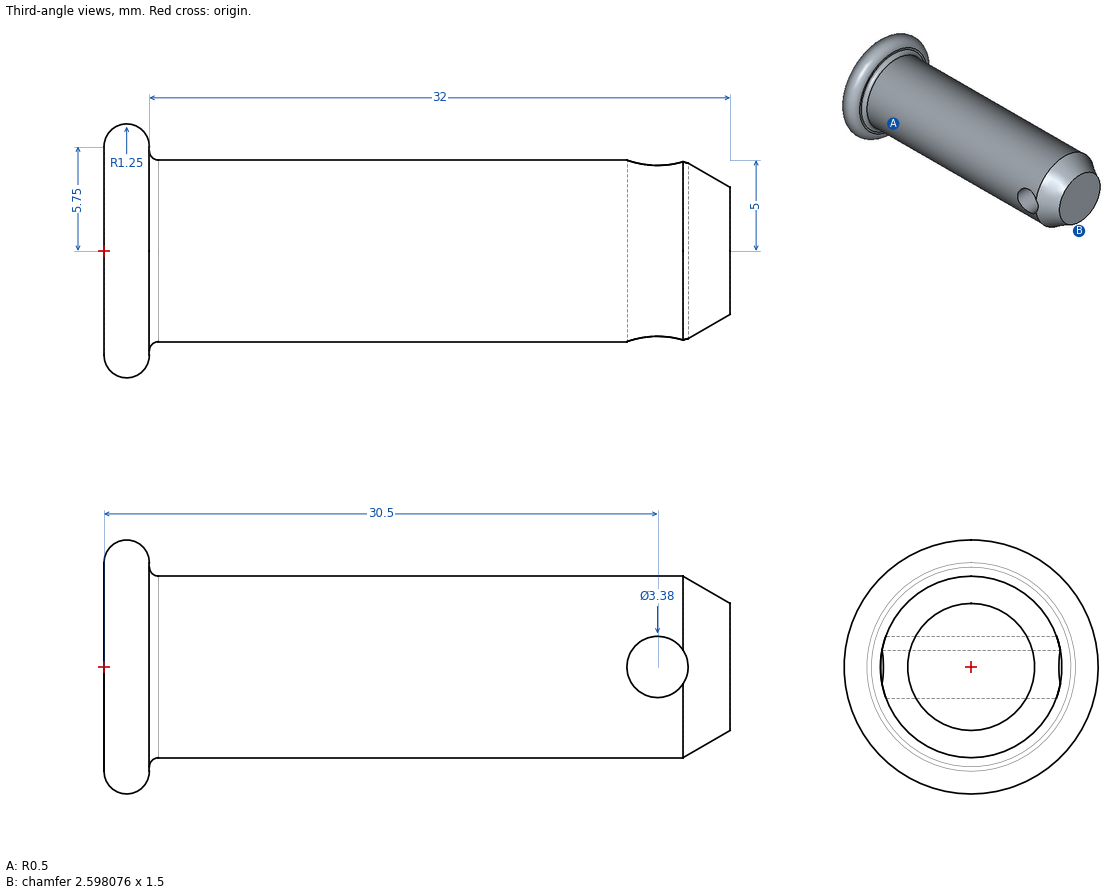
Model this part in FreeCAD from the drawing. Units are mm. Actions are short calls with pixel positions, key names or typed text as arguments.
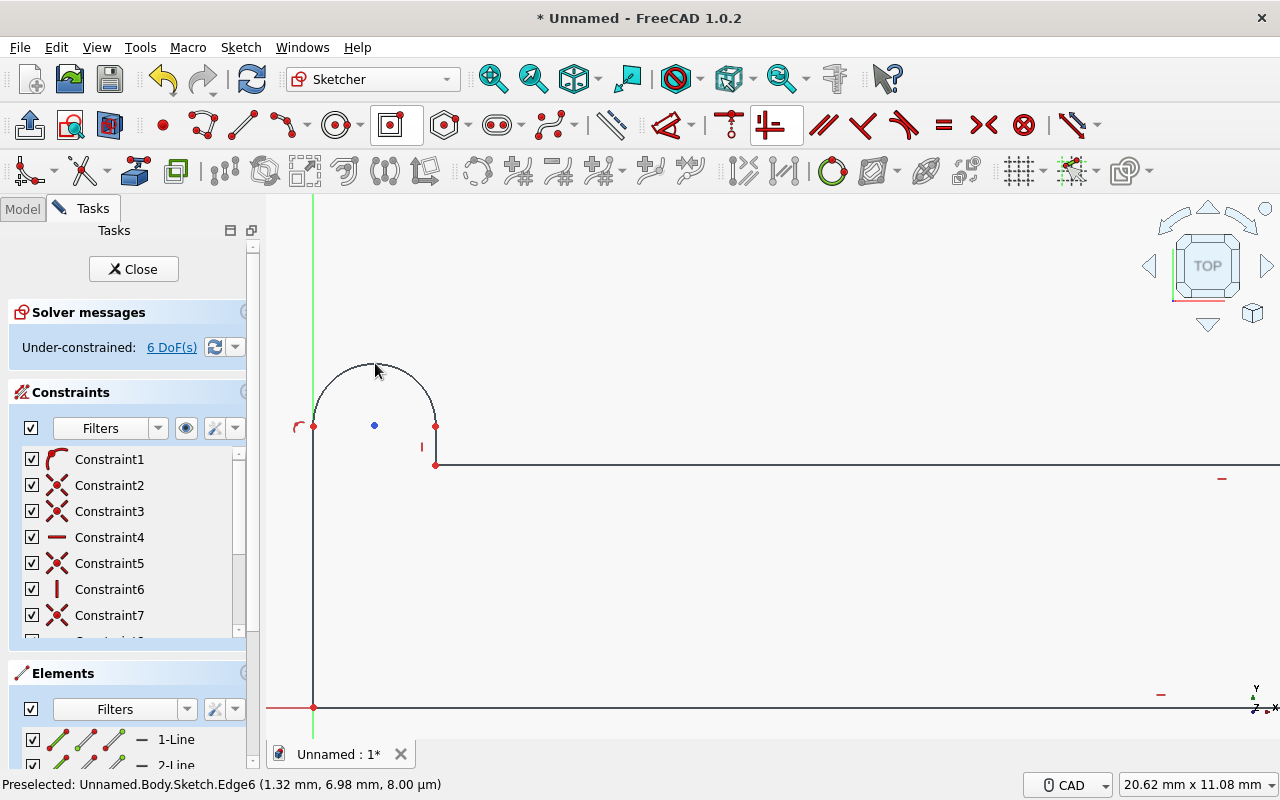
click(313, 511)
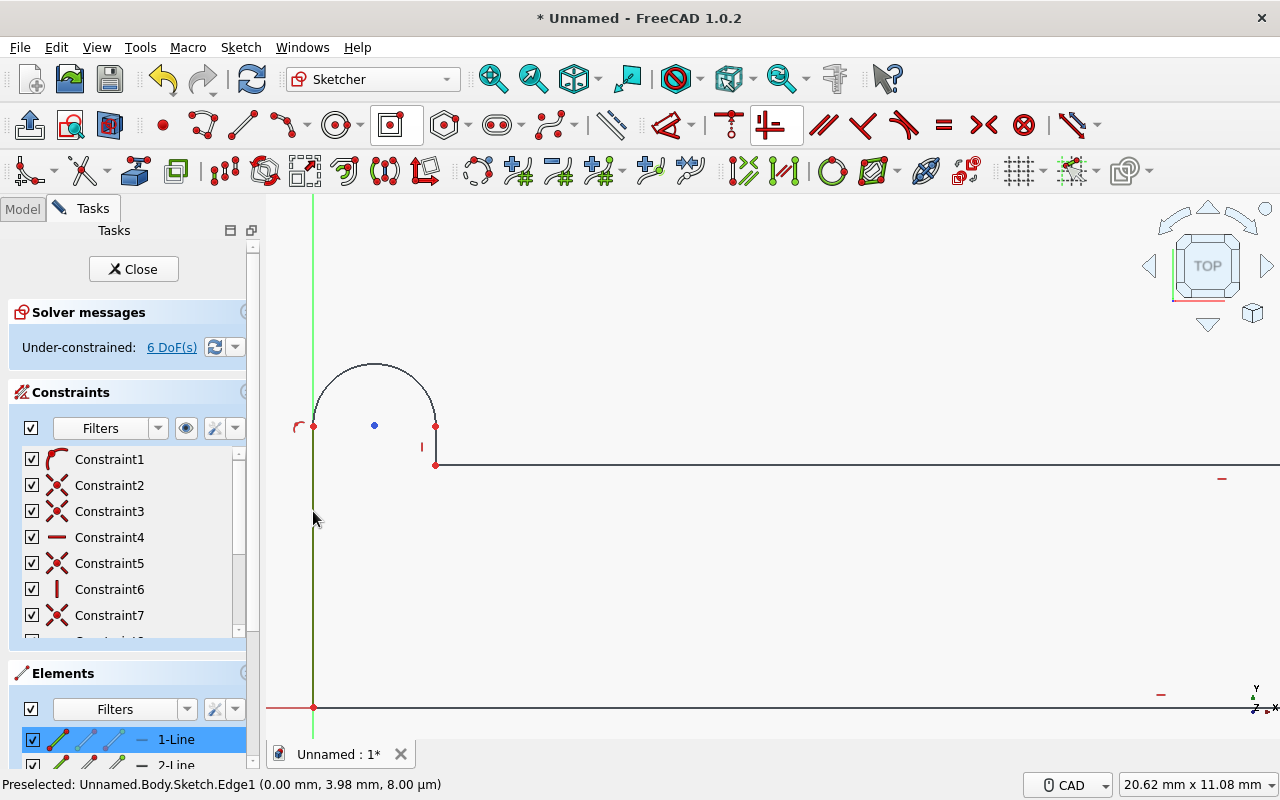
click(411, 376)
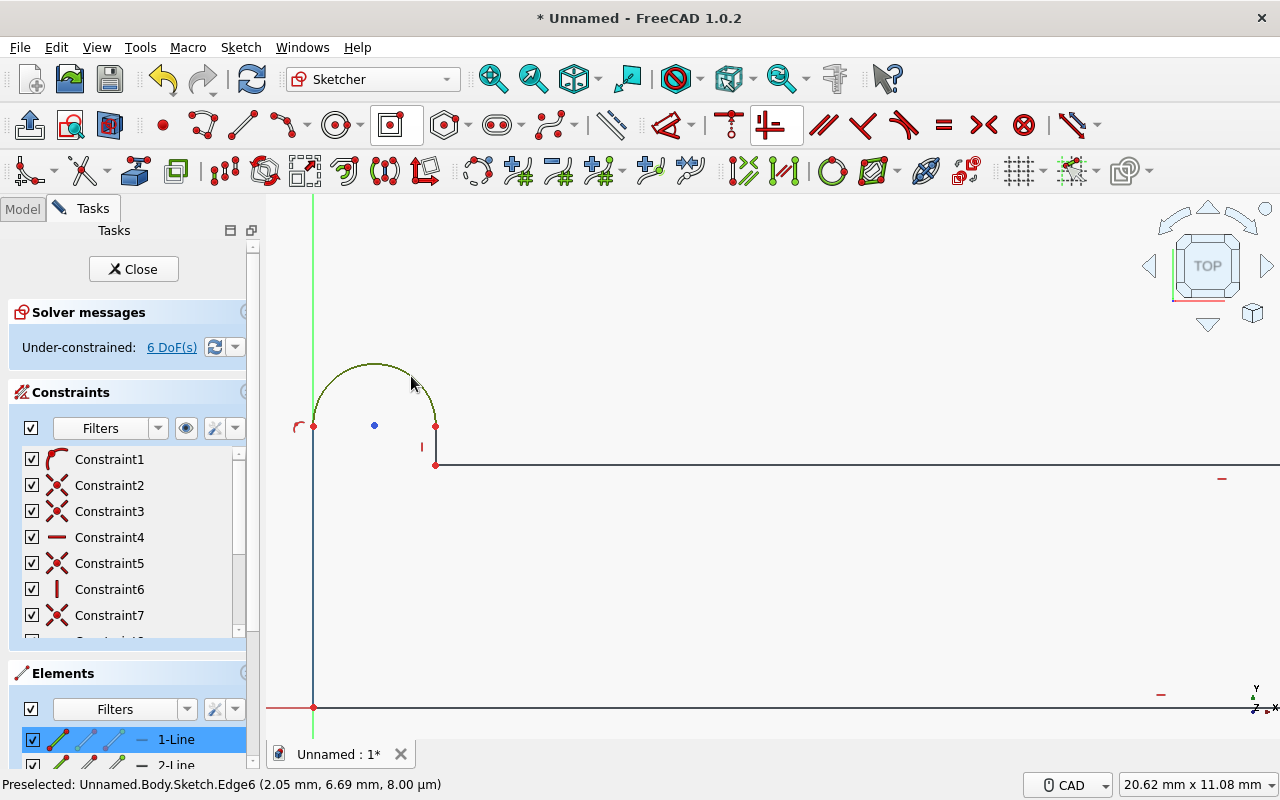
key(t)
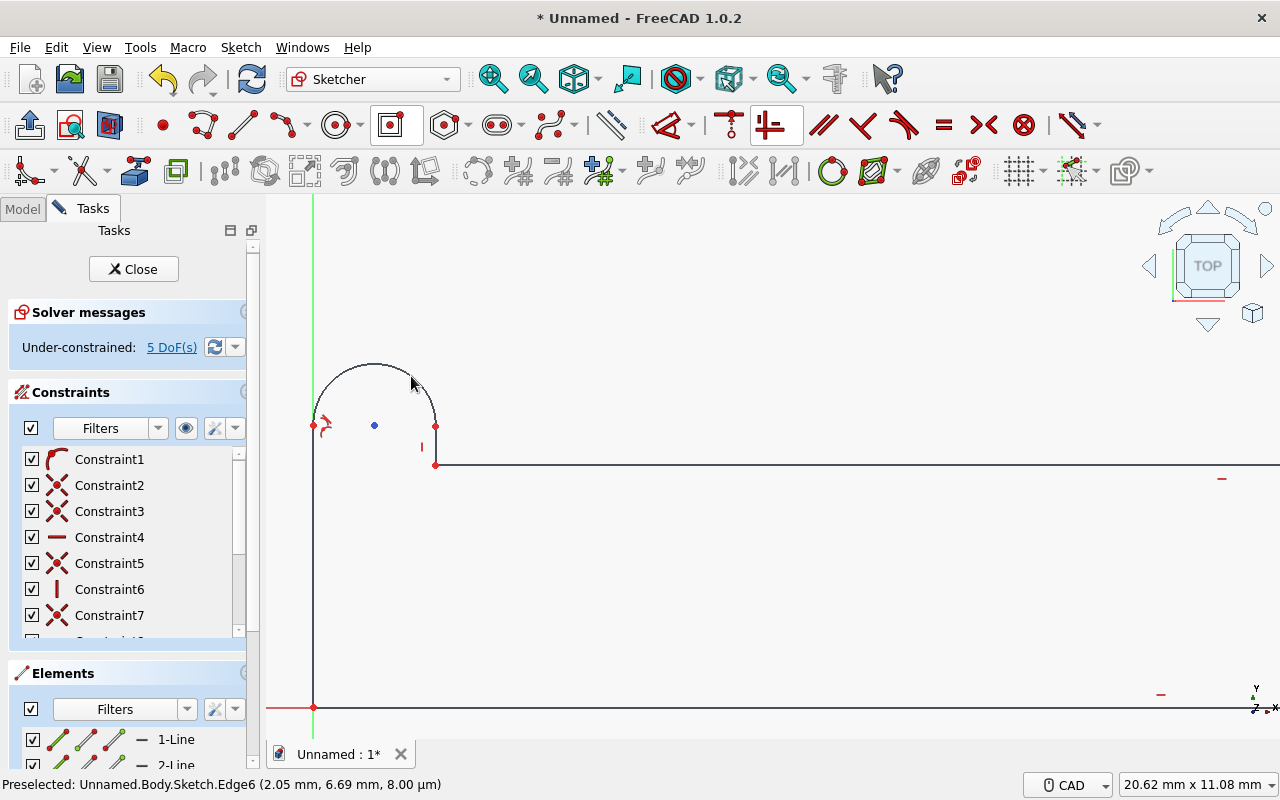
click(436, 454)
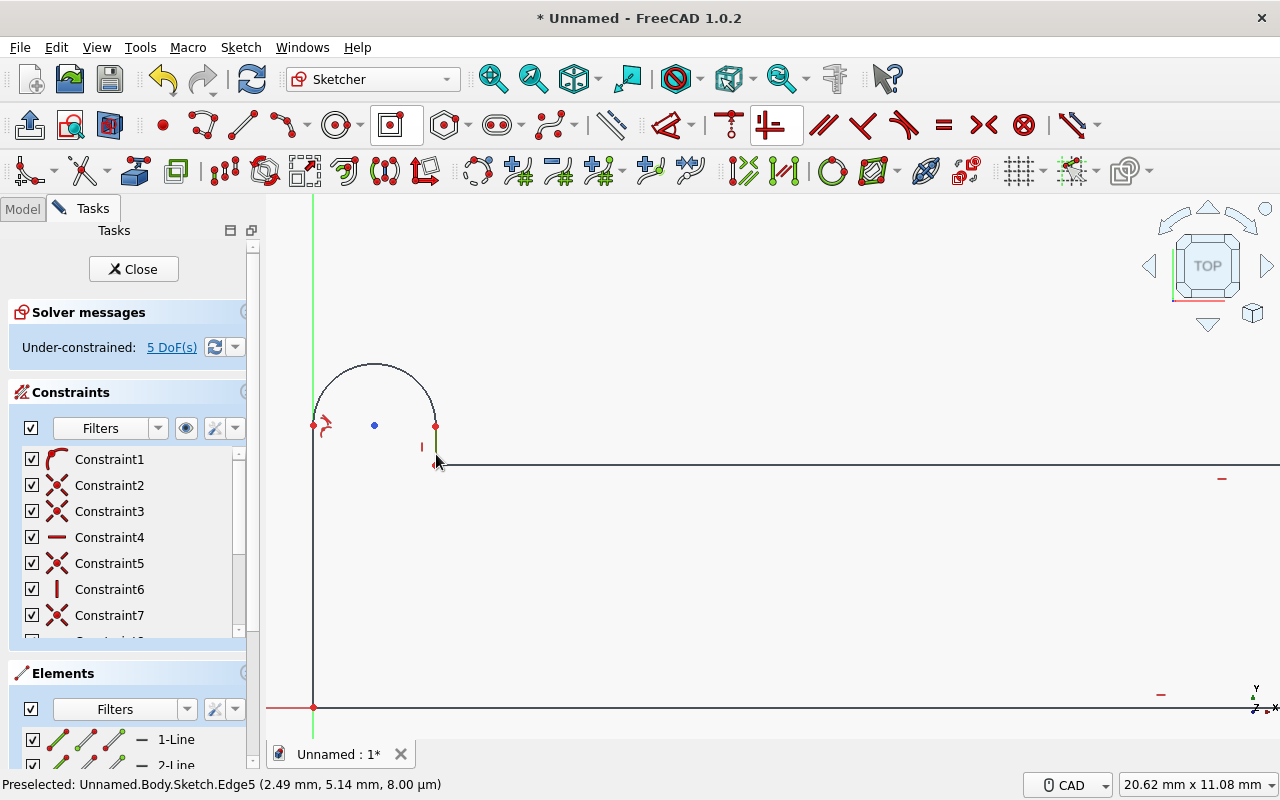
click(411, 376)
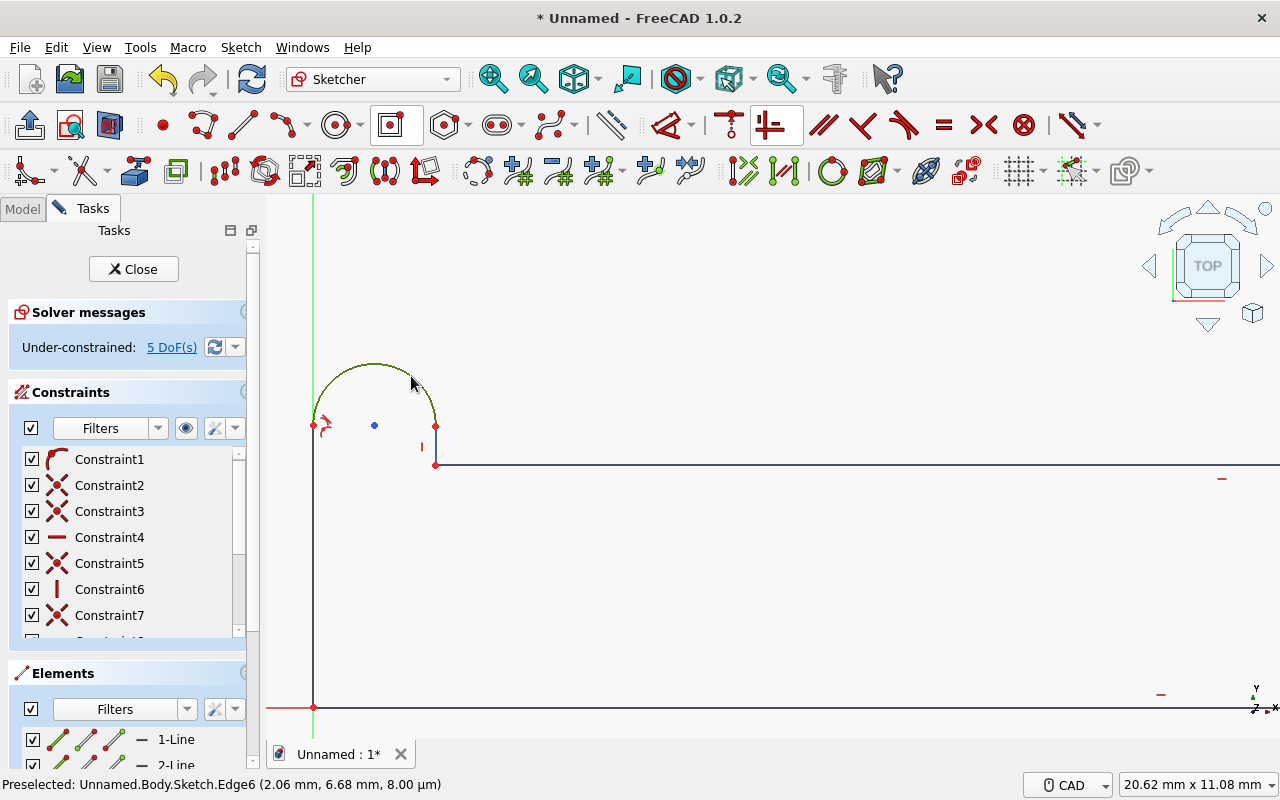
key(t)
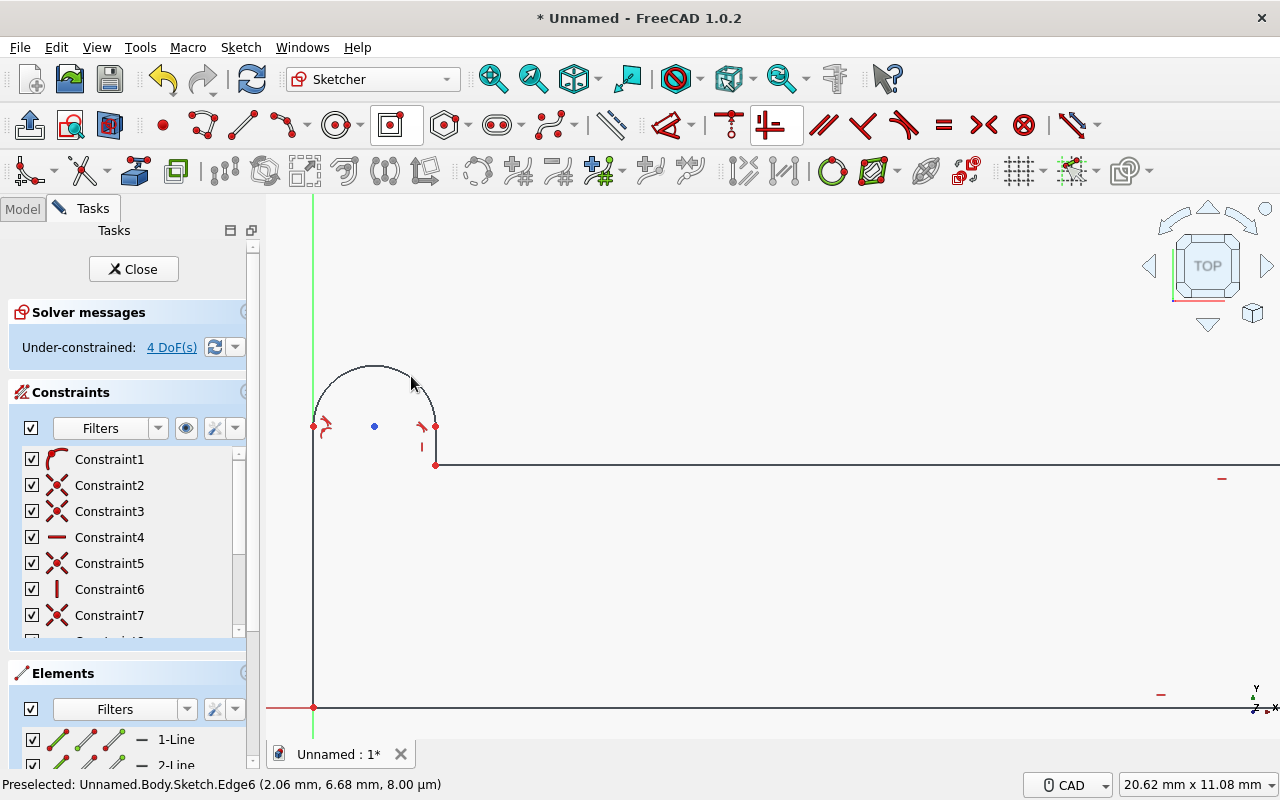
click(410, 377)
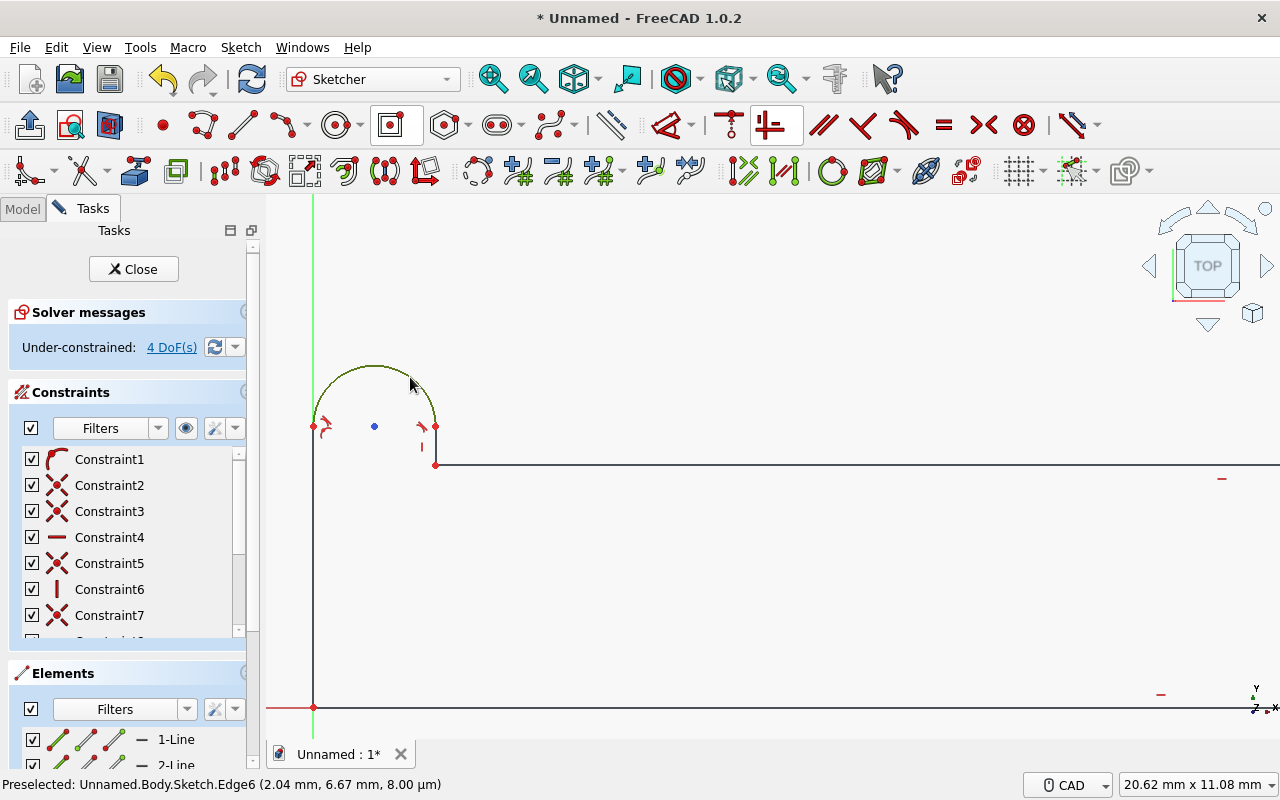
key(k)
key(r)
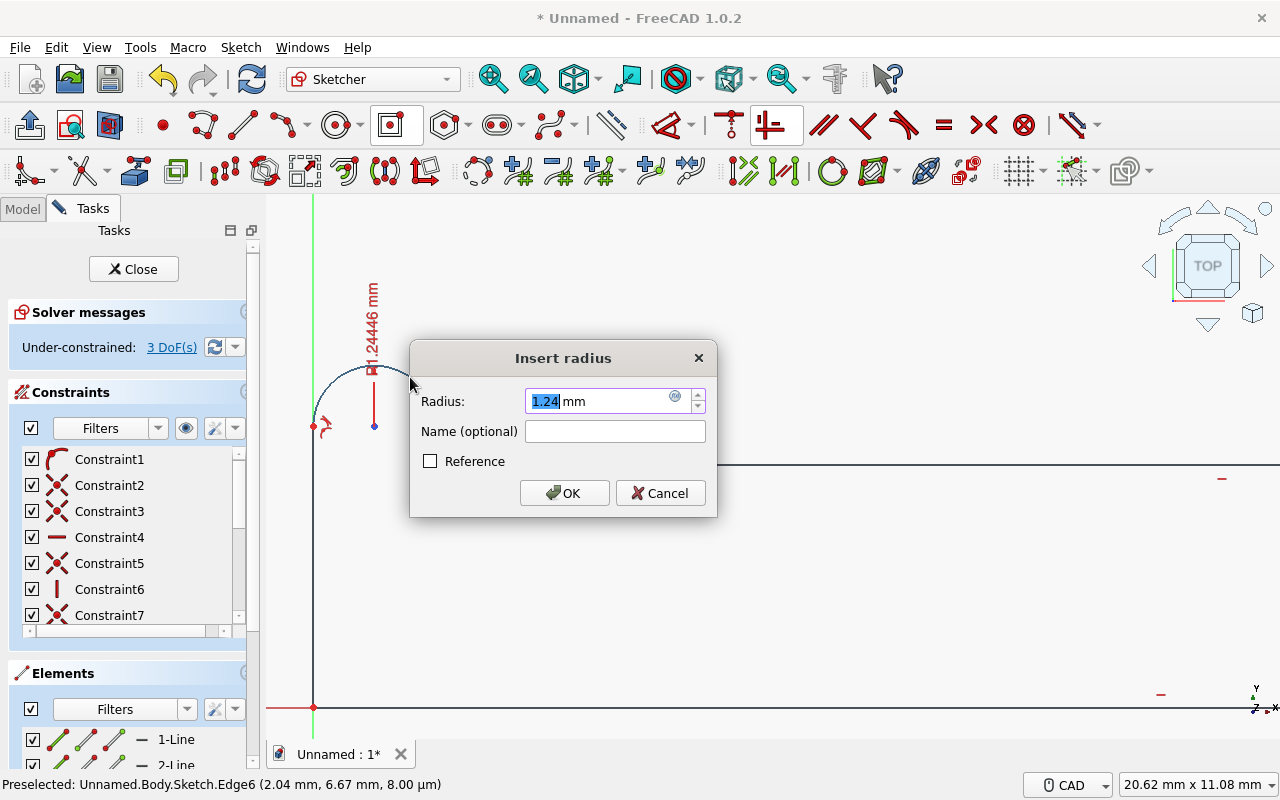
text(1.25)
key(Return)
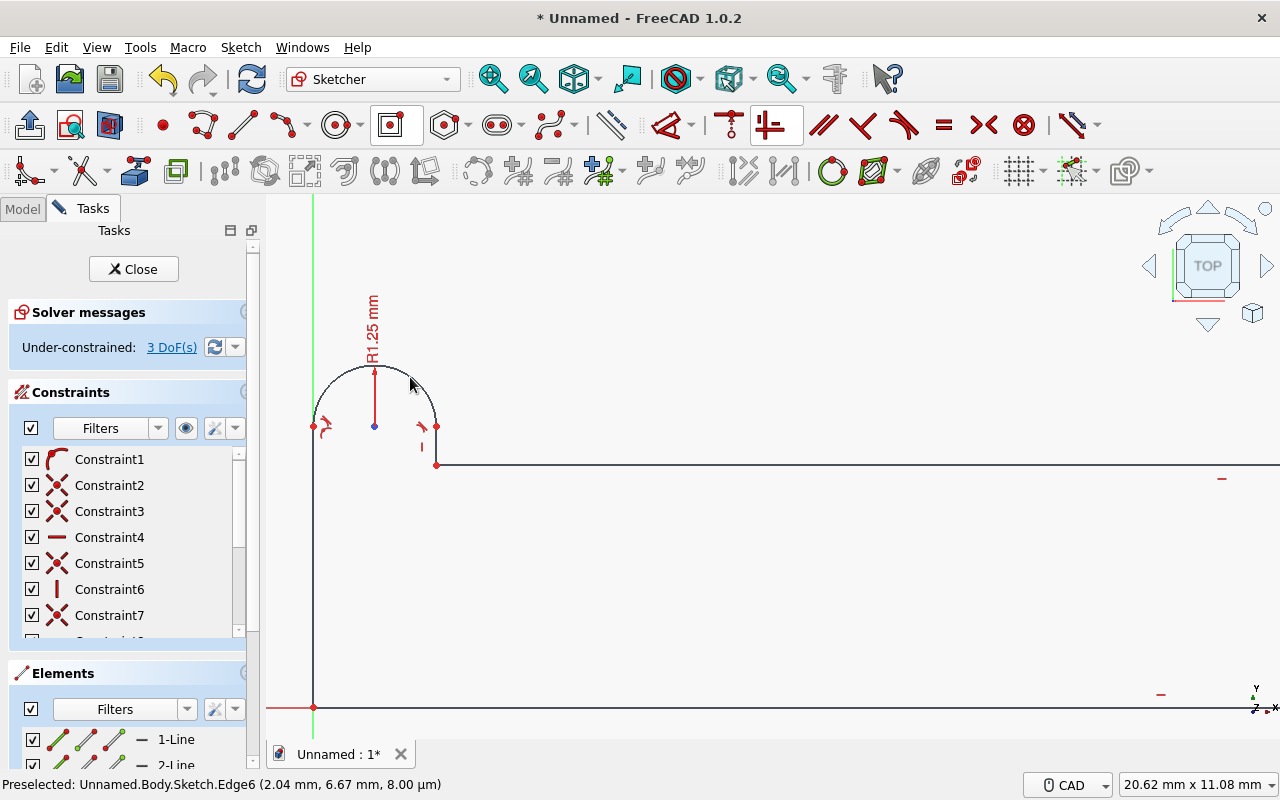
scroll(438, 426, down, 5)